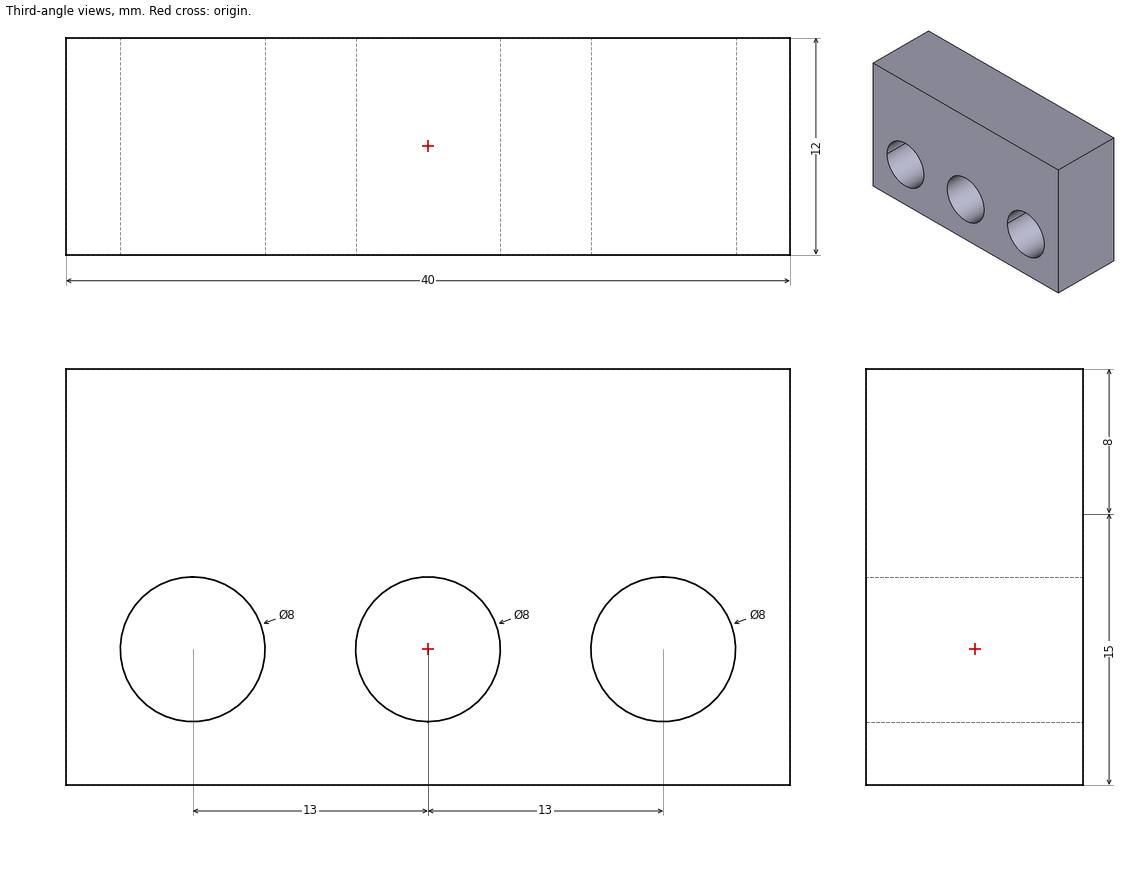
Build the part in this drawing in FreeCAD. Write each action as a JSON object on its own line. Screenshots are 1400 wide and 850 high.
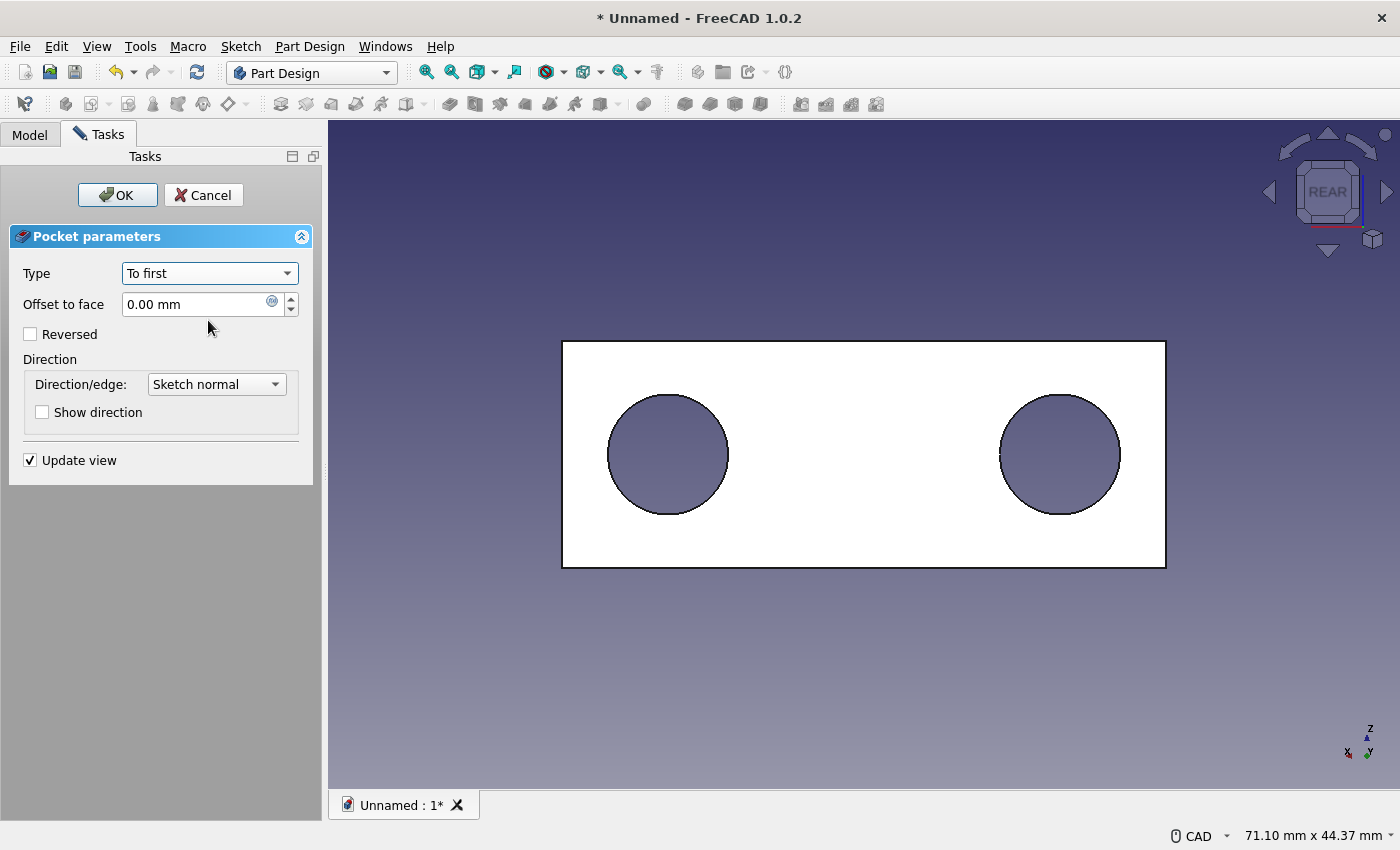
{"action": "left_click", "coordinate": [118, 195]}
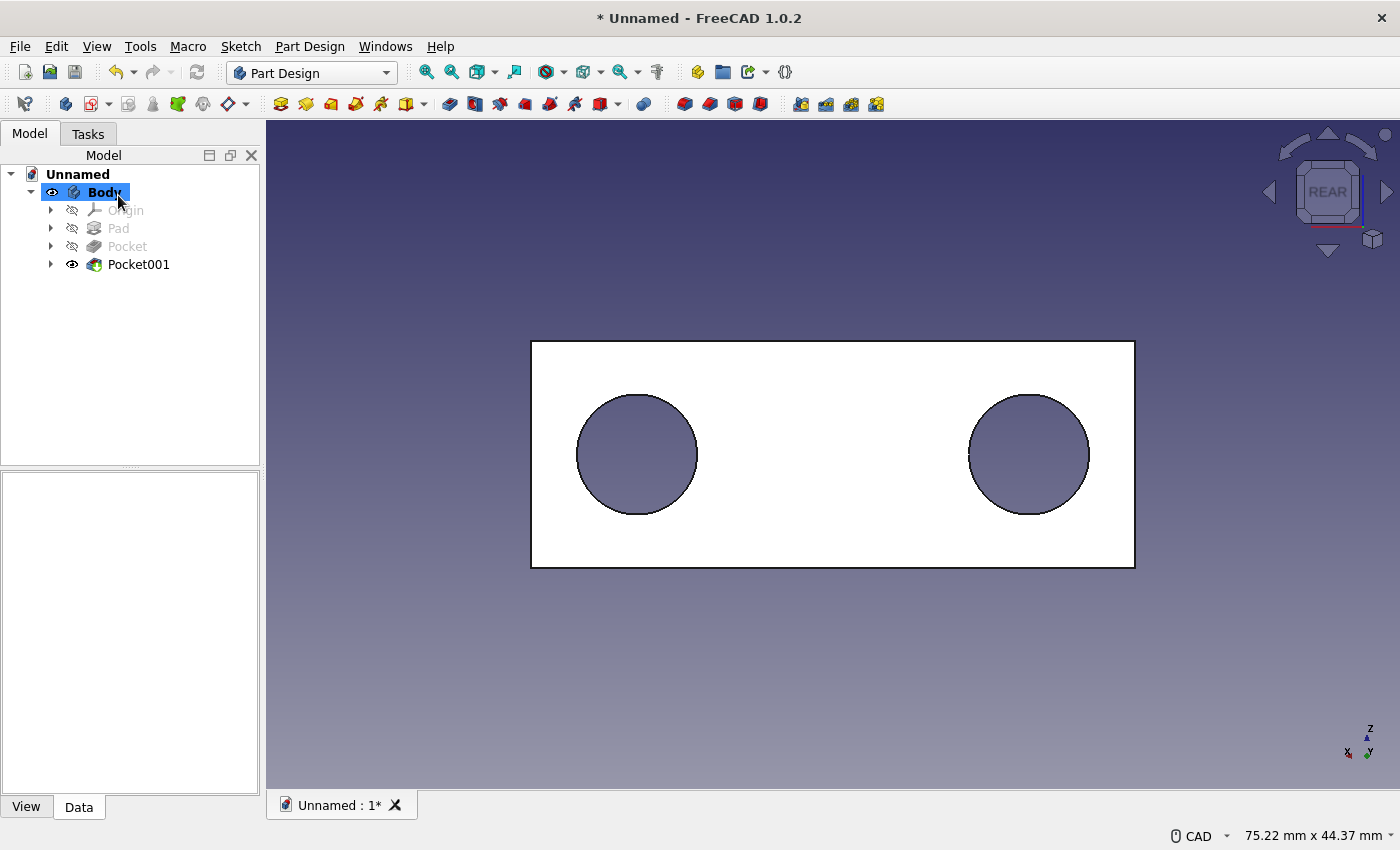
{"action": "key", "text": "0"}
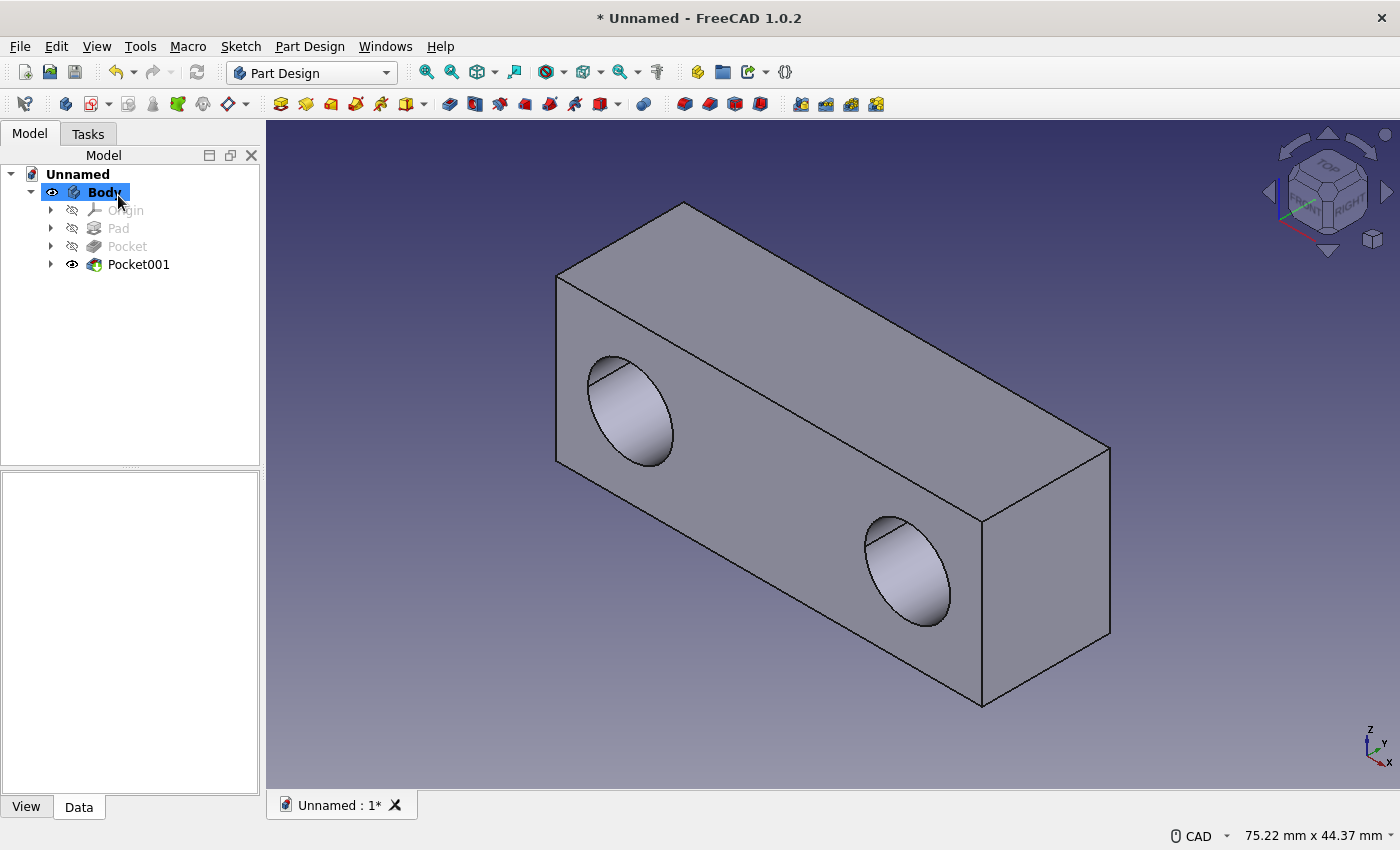
{"action": "left_click", "coordinate": [769, 490]}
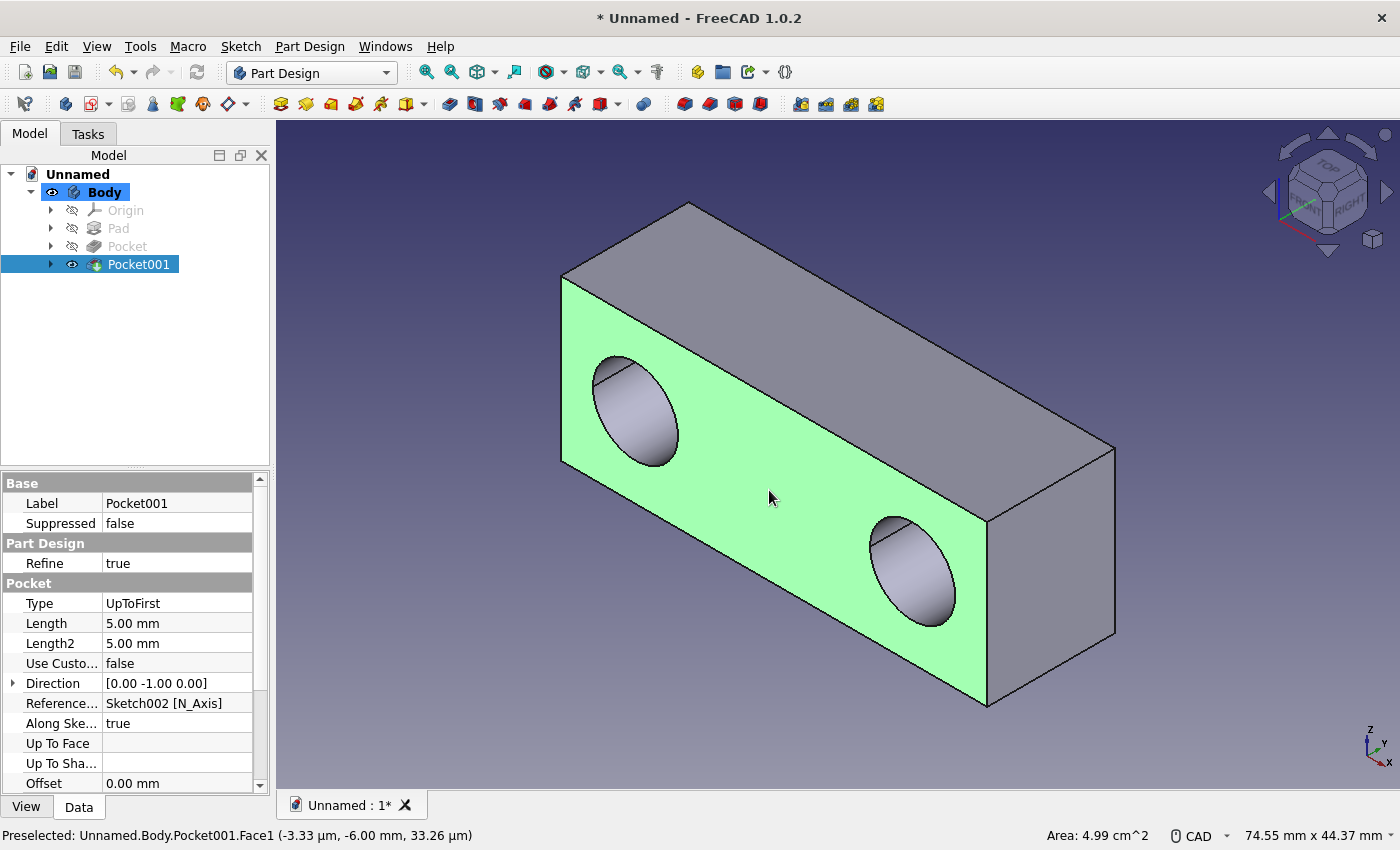
{"action": "left_click", "coordinate": [90, 104]}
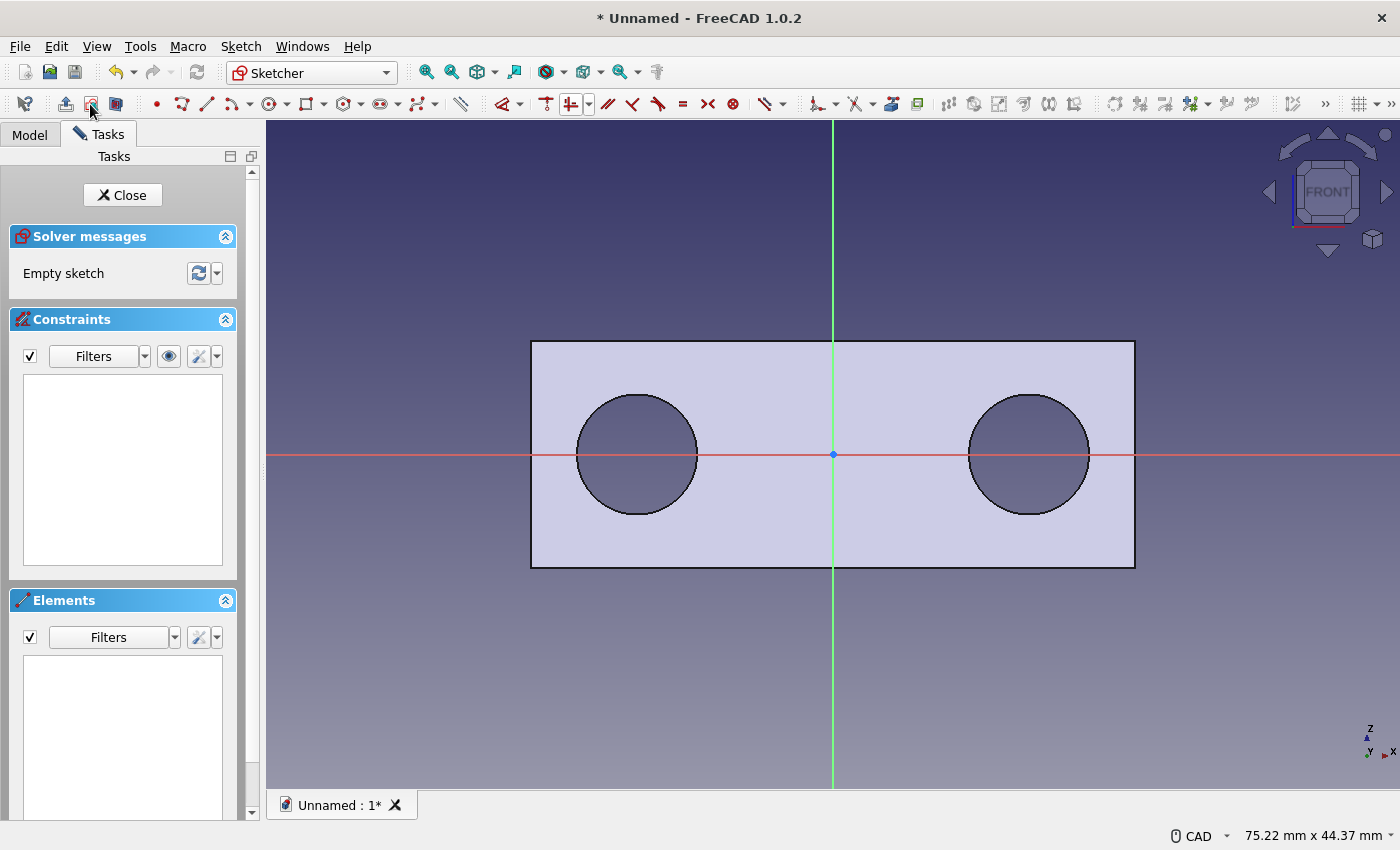
{"action": "scroll", "coordinate": [863, 455], "scroll_direction": "up", "scroll_amount": 6}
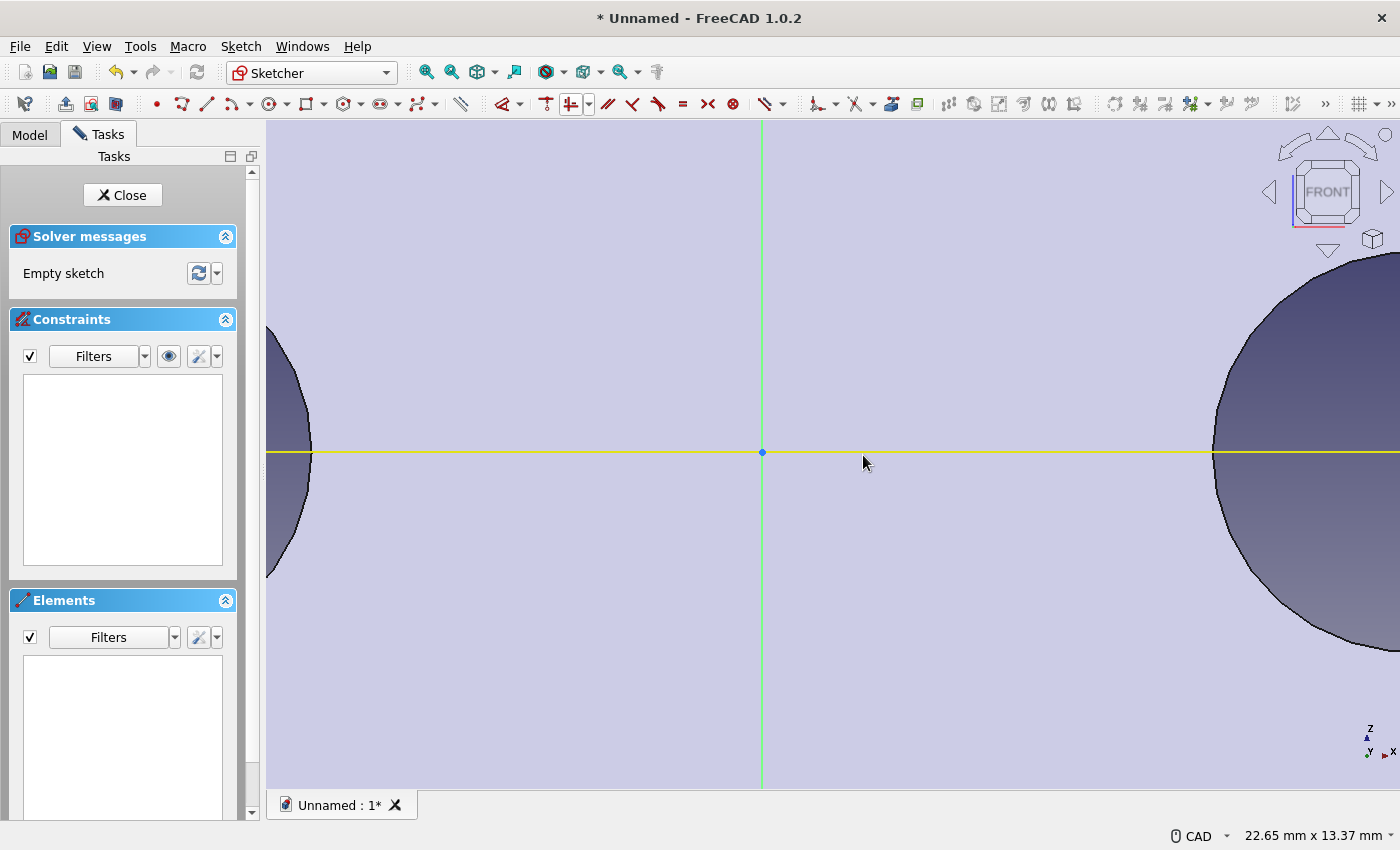
{"action": "left_click", "coordinate": [268, 104]}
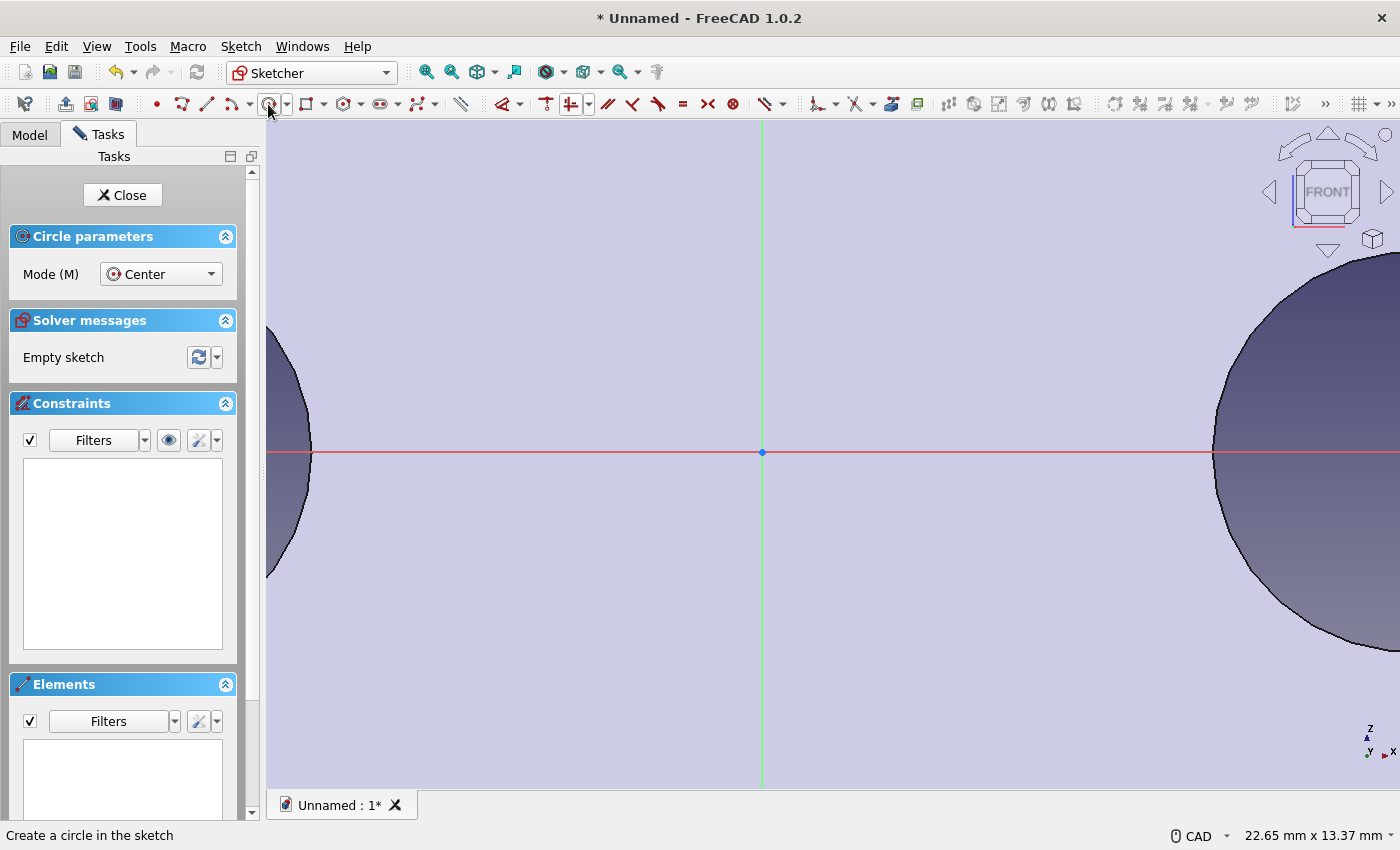
{"action": "left_click", "coordinate": [762, 452]}
{"action": "left_click", "coordinate": [904, 311]}
{"action": "key", "text": "Escape"}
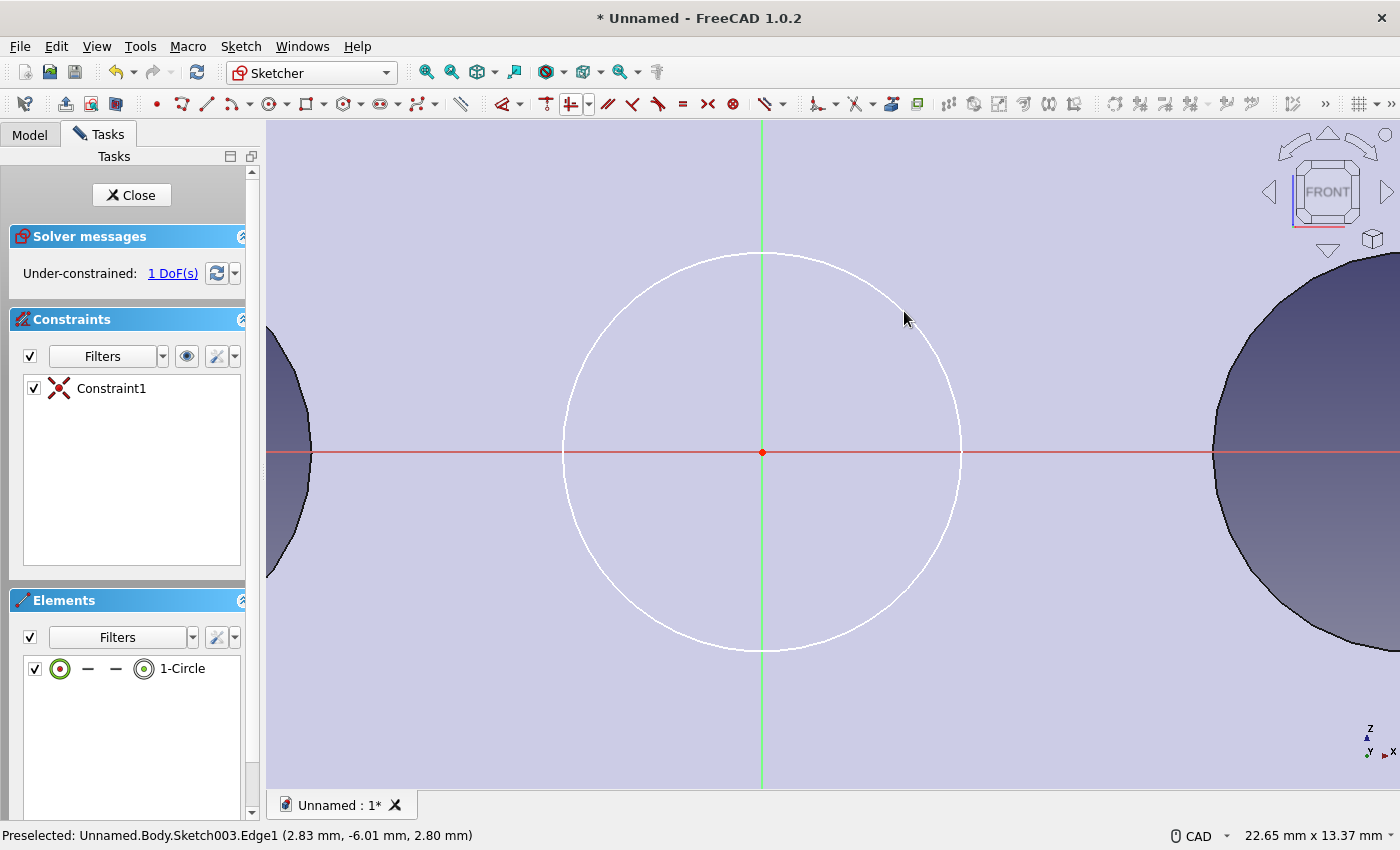
{"action": "key", "text": "d"}